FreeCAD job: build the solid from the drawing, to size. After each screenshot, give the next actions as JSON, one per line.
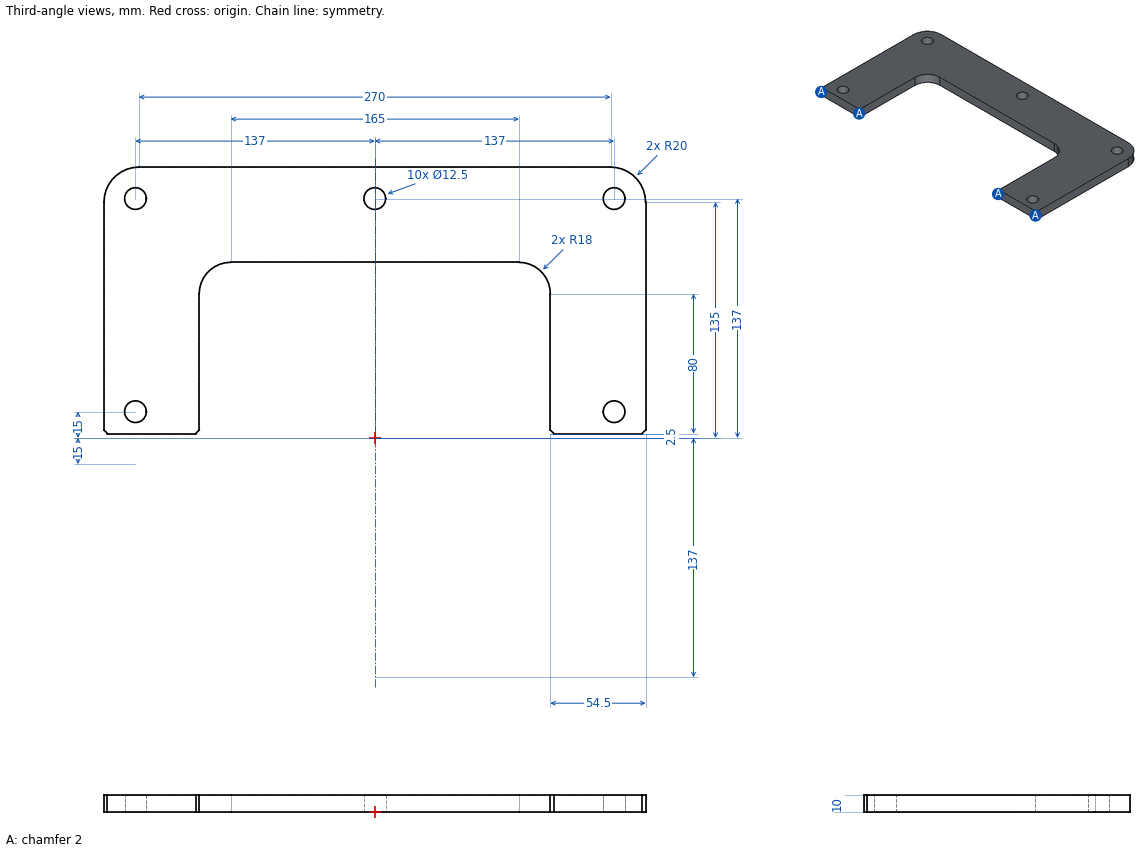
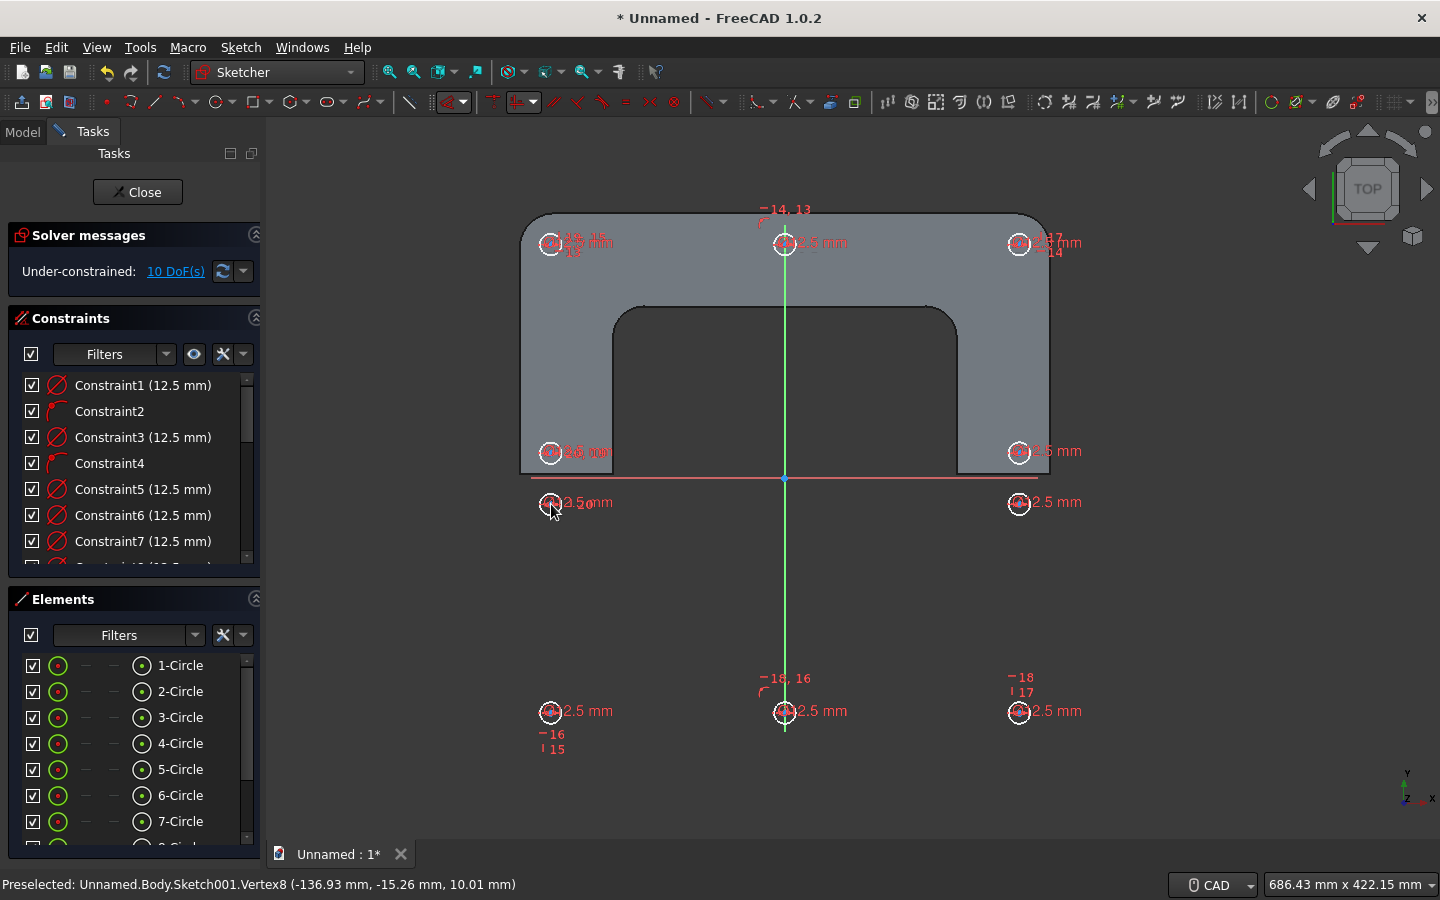
{"action": "left_click", "coordinate": [1019, 713]}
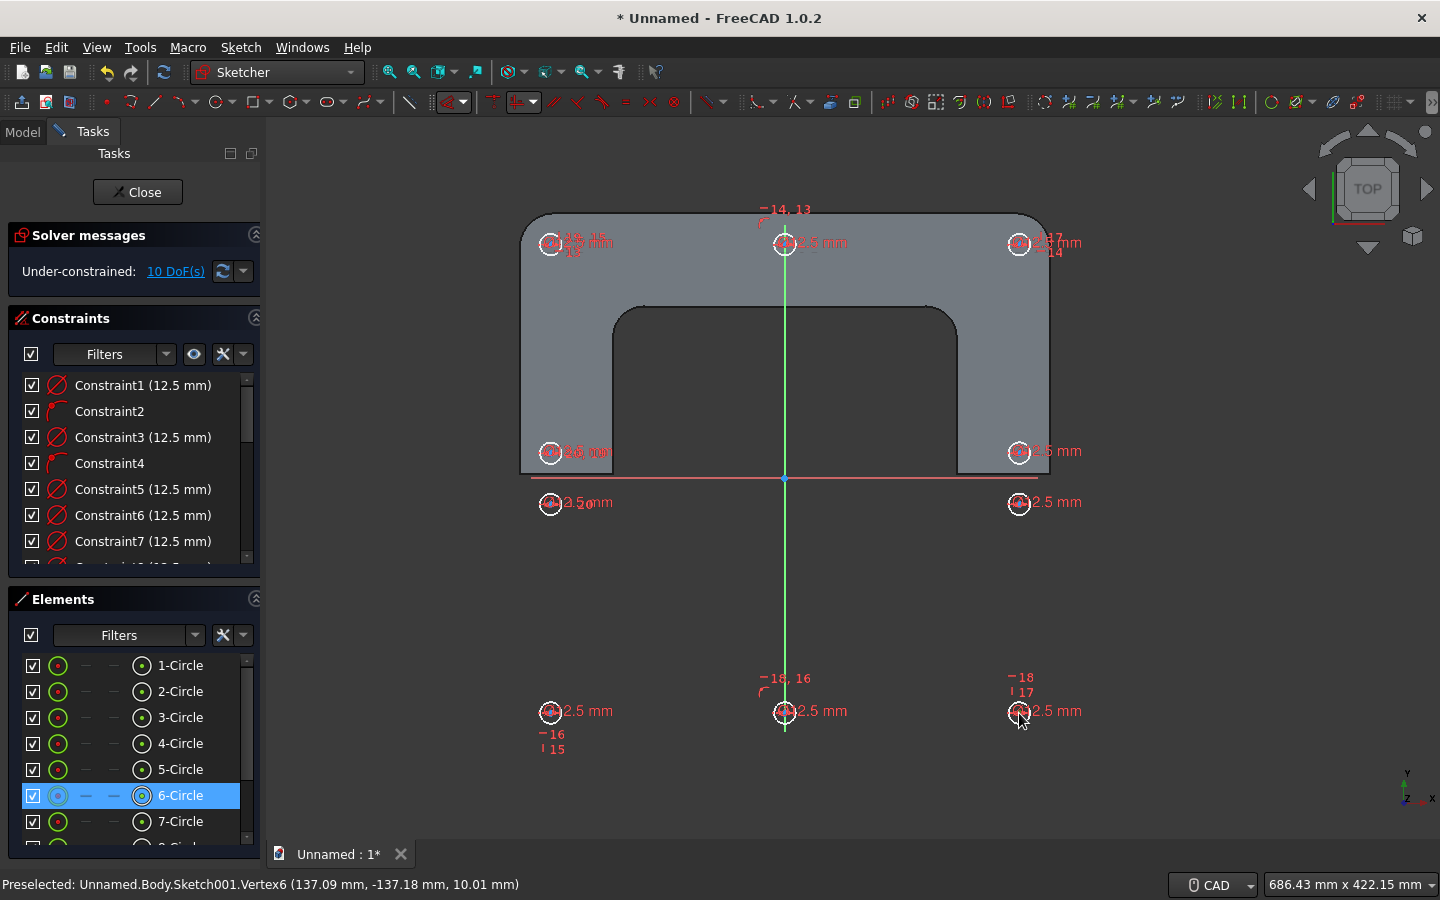
{"action": "left_click", "coordinate": [1019, 504]}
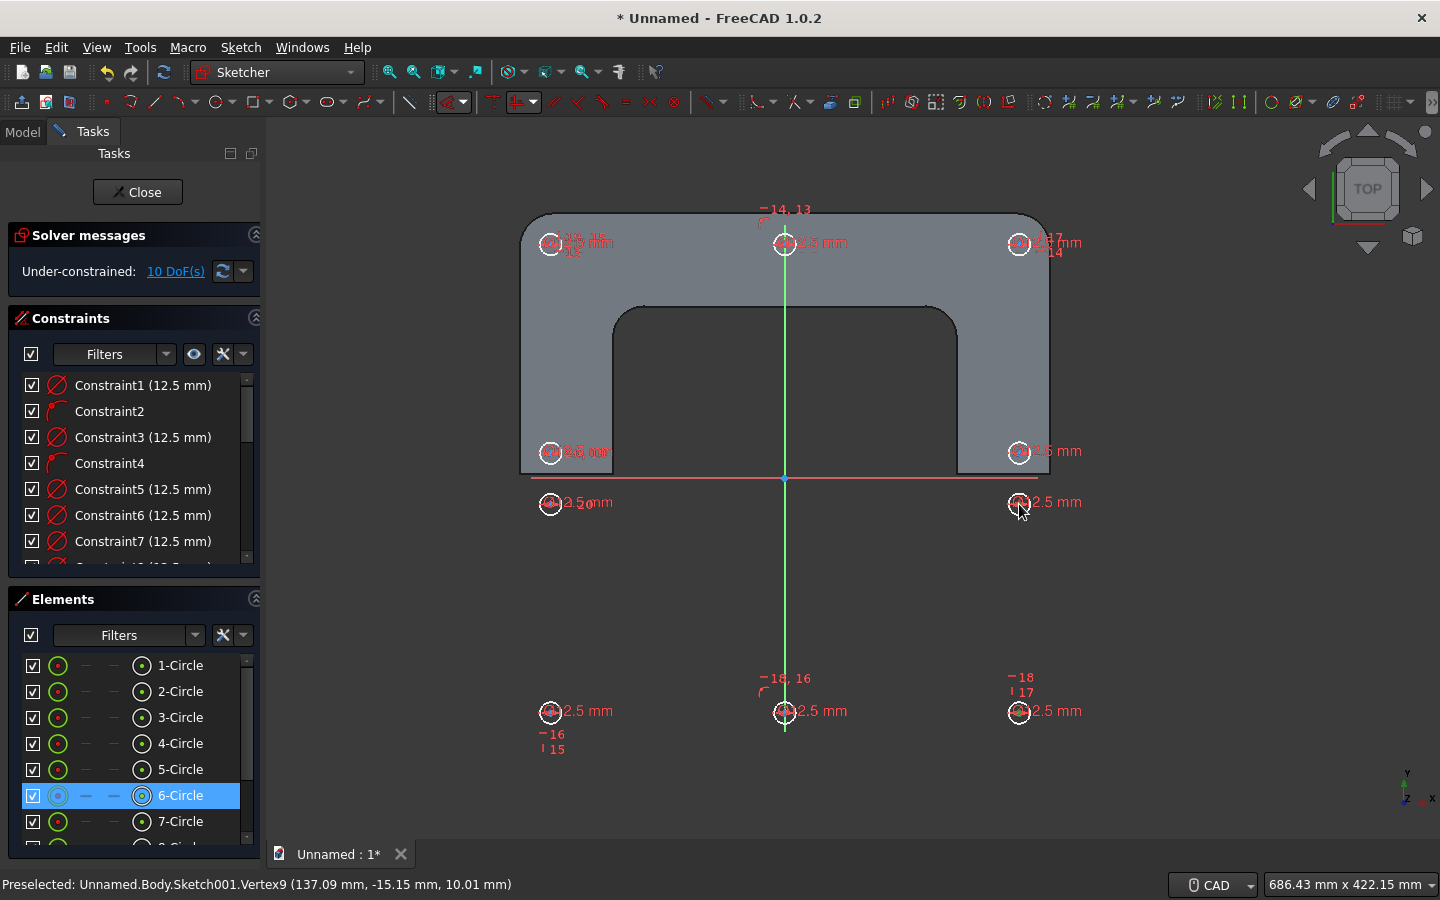
{"action": "key", "text": "v"}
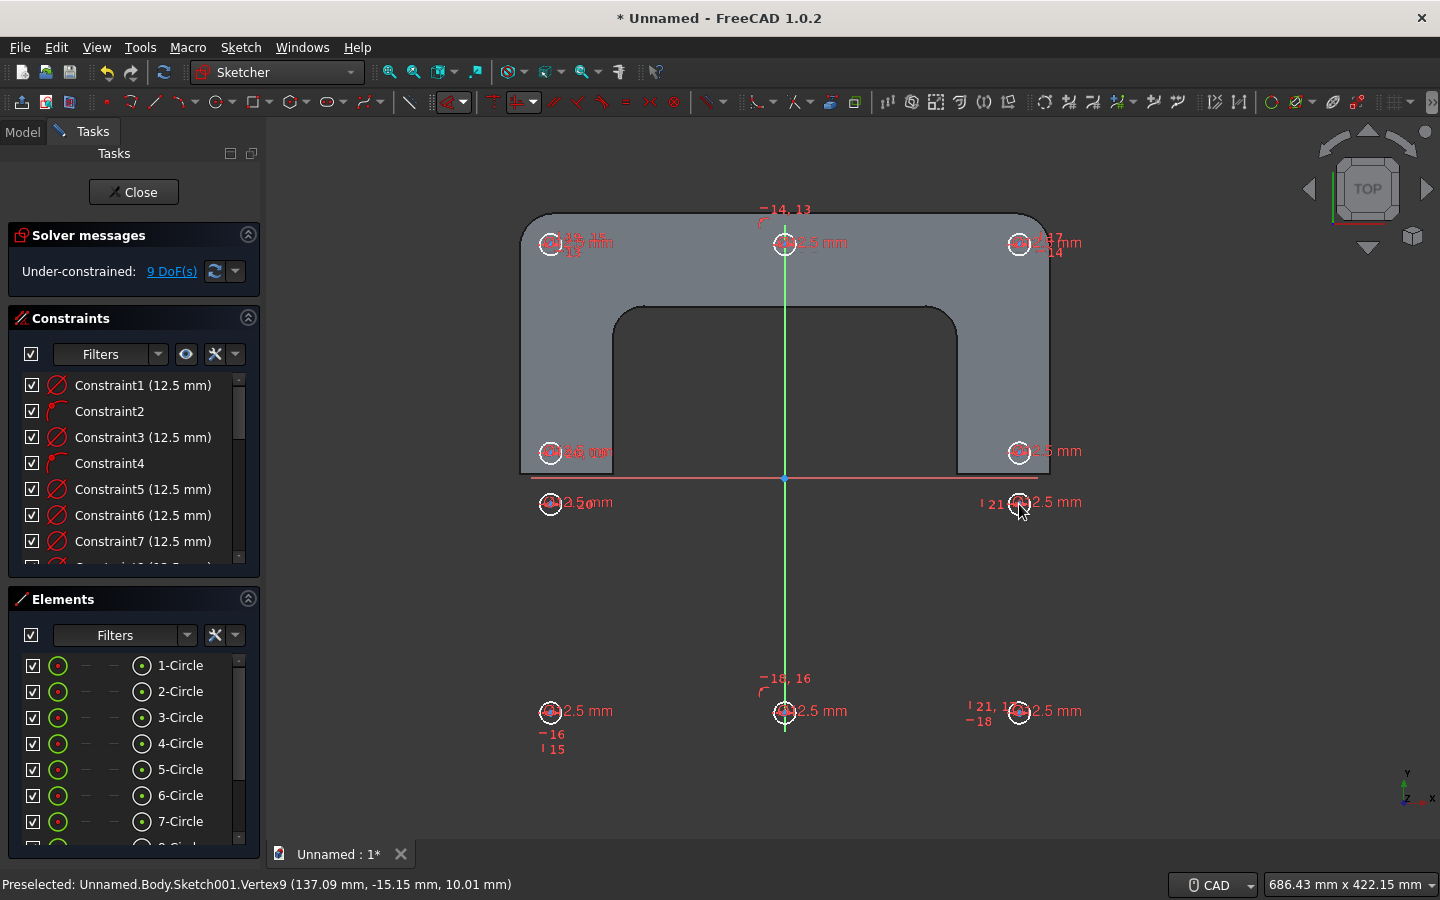
{"action": "left_click", "coordinate": [551, 504]}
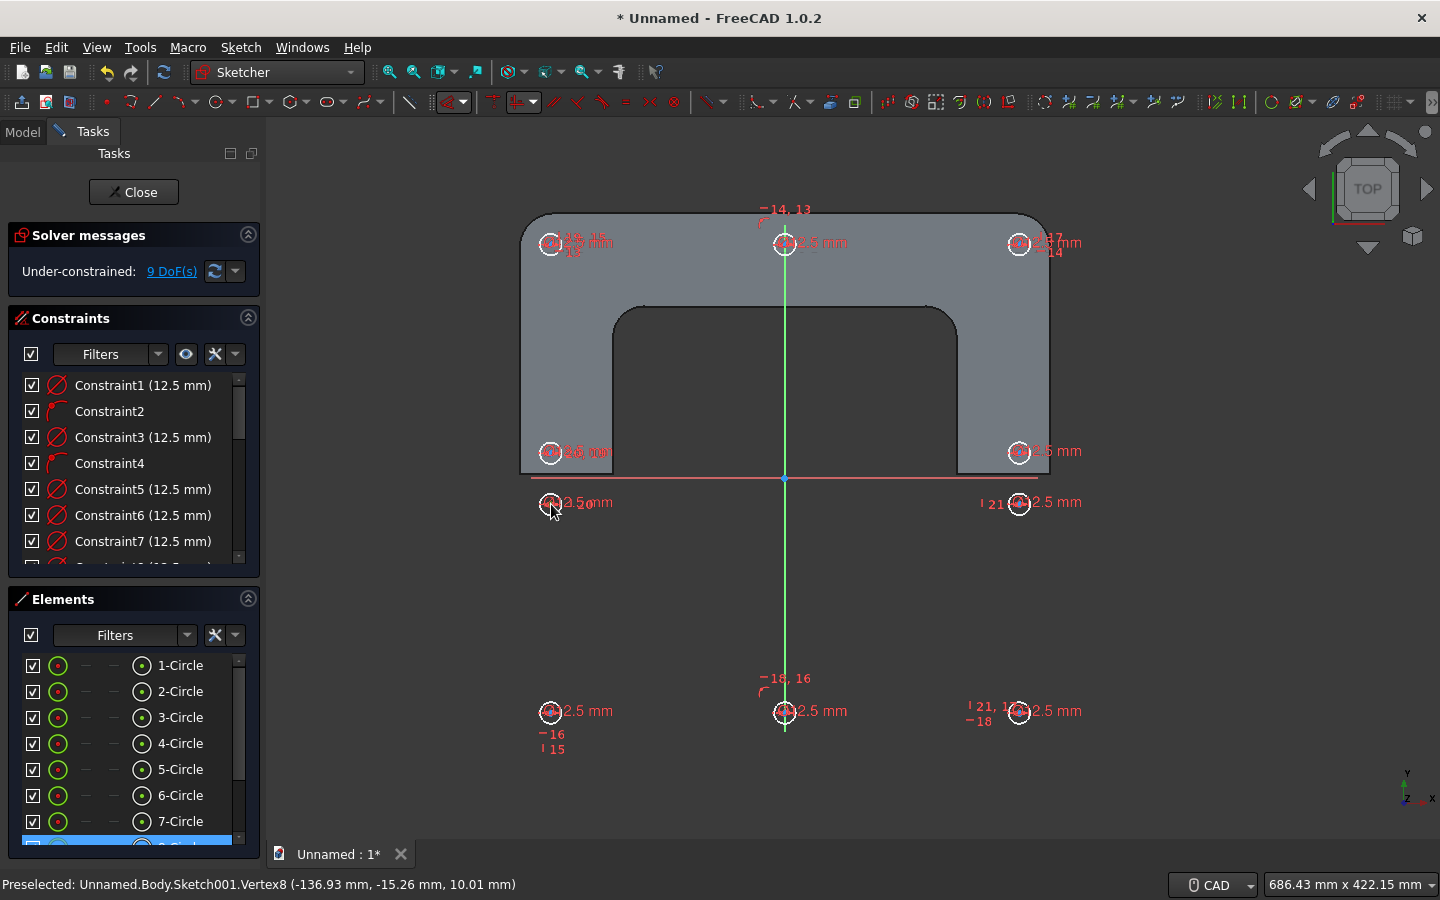
{"action": "left_click", "coordinate": [1019, 504]}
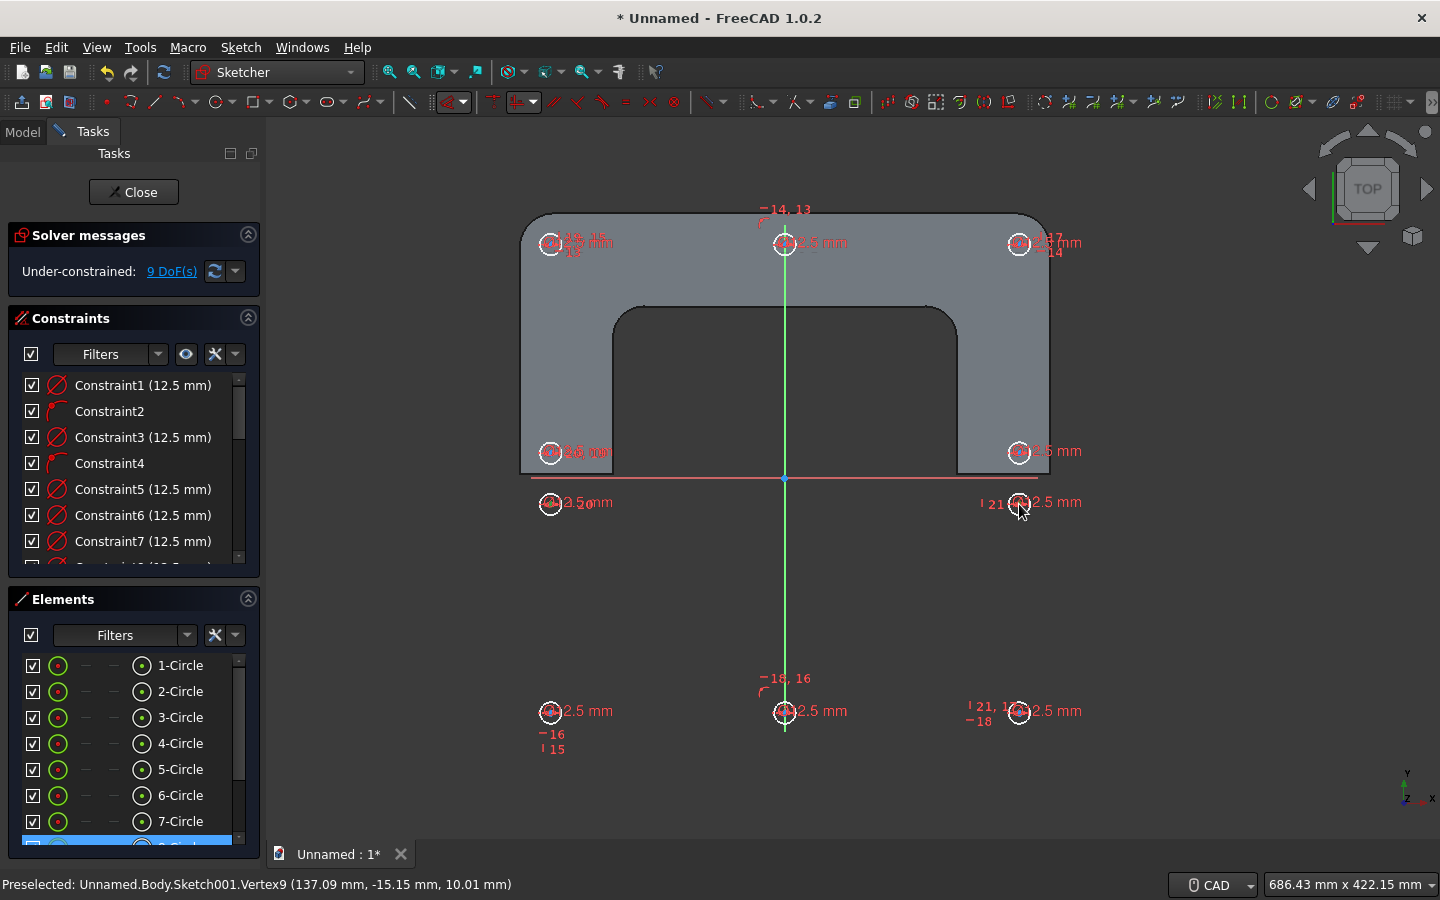
{"action": "key", "text": "h"}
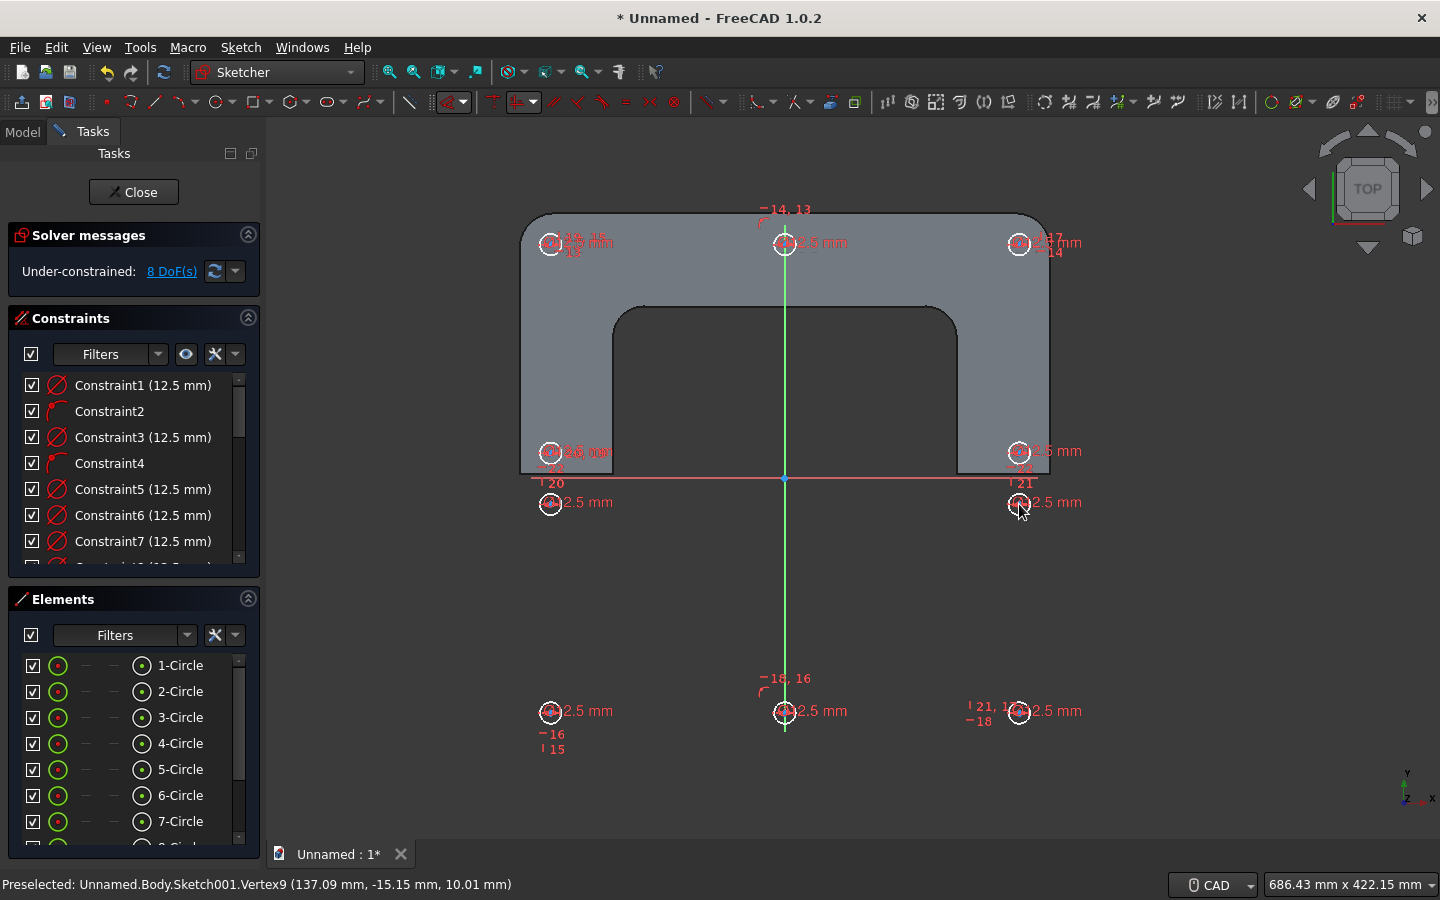
{"action": "left_click", "coordinate": [1019, 504]}